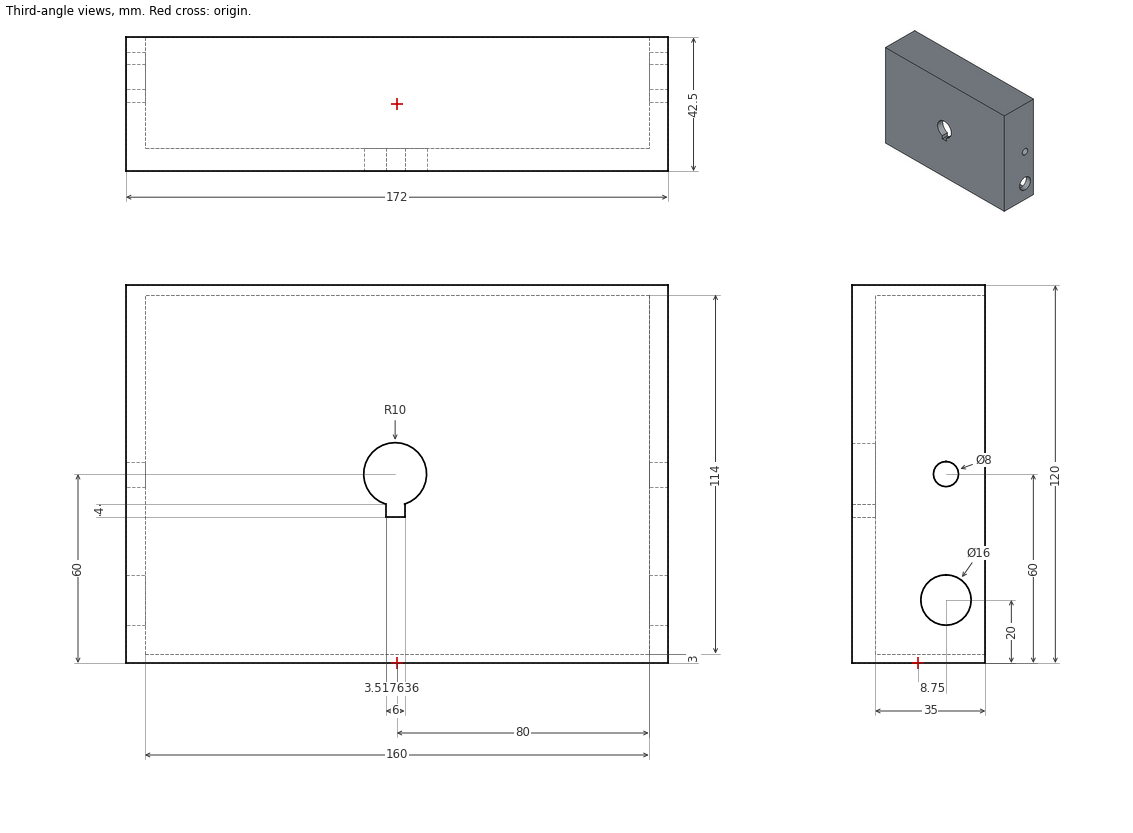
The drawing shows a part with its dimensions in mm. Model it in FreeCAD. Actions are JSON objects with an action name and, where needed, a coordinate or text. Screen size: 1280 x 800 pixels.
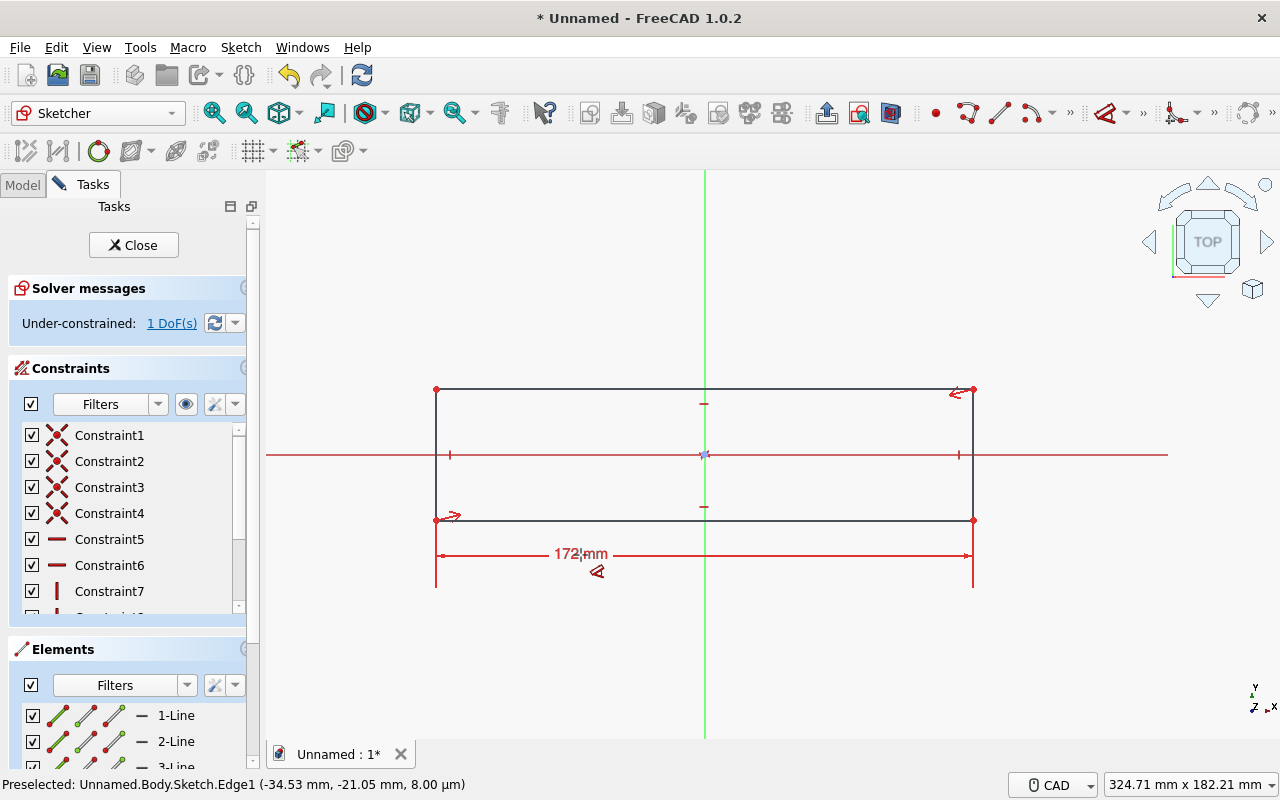
{"action": "left_click", "coordinate": [973, 481]}
{"action": "left_click", "coordinate": [1007, 425]}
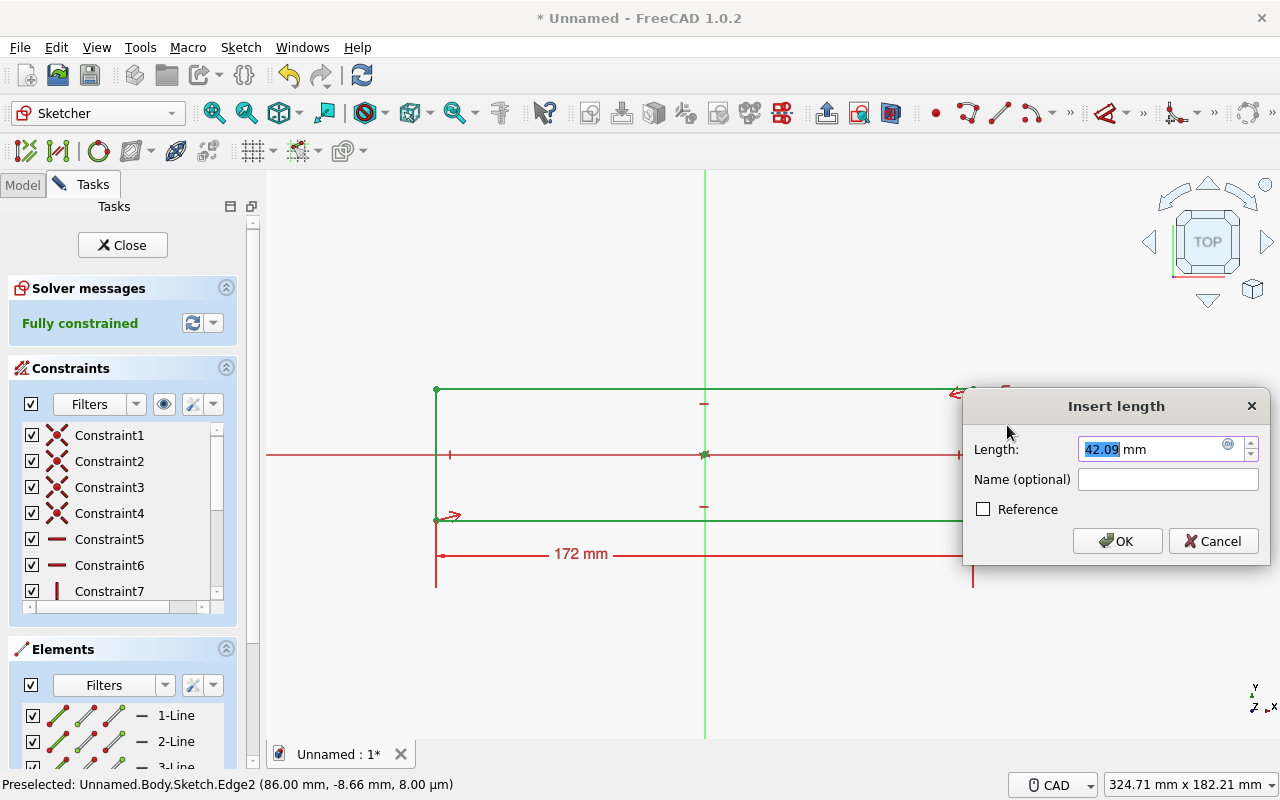
{"action": "type", "text": "42.5"}
{"action": "key", "text": "Return"}
{"action": "key", "text": "Escape"}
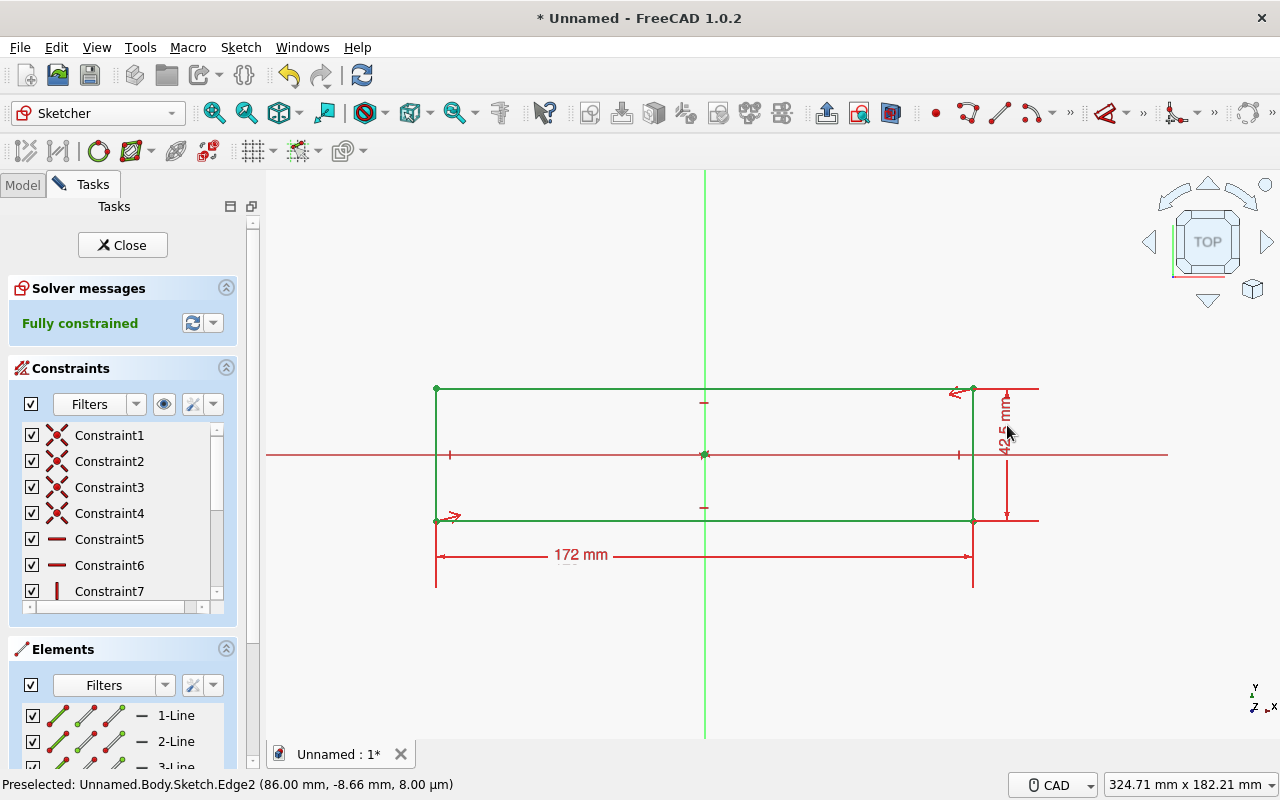
{"action": "left_click", "coordinate": [123, 245]}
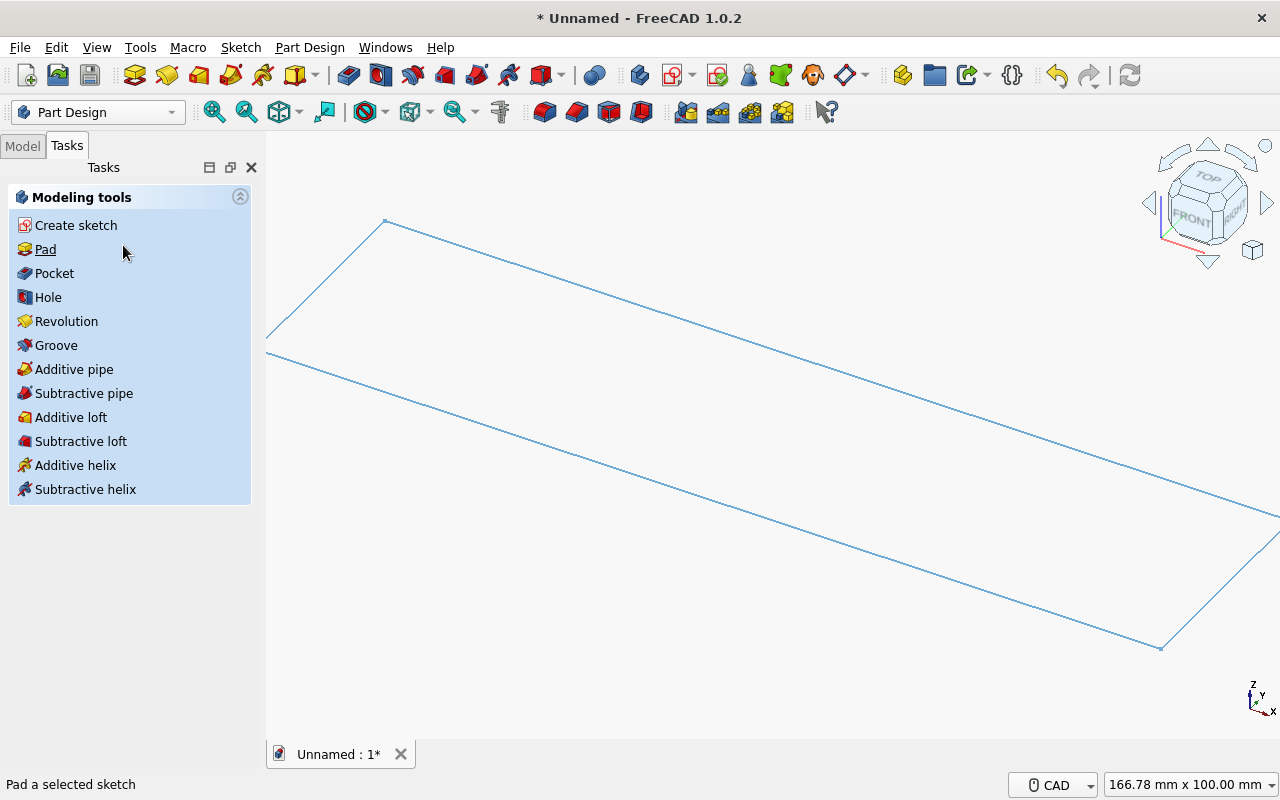
{"action": "left_click", "coordinate": [136, 76]}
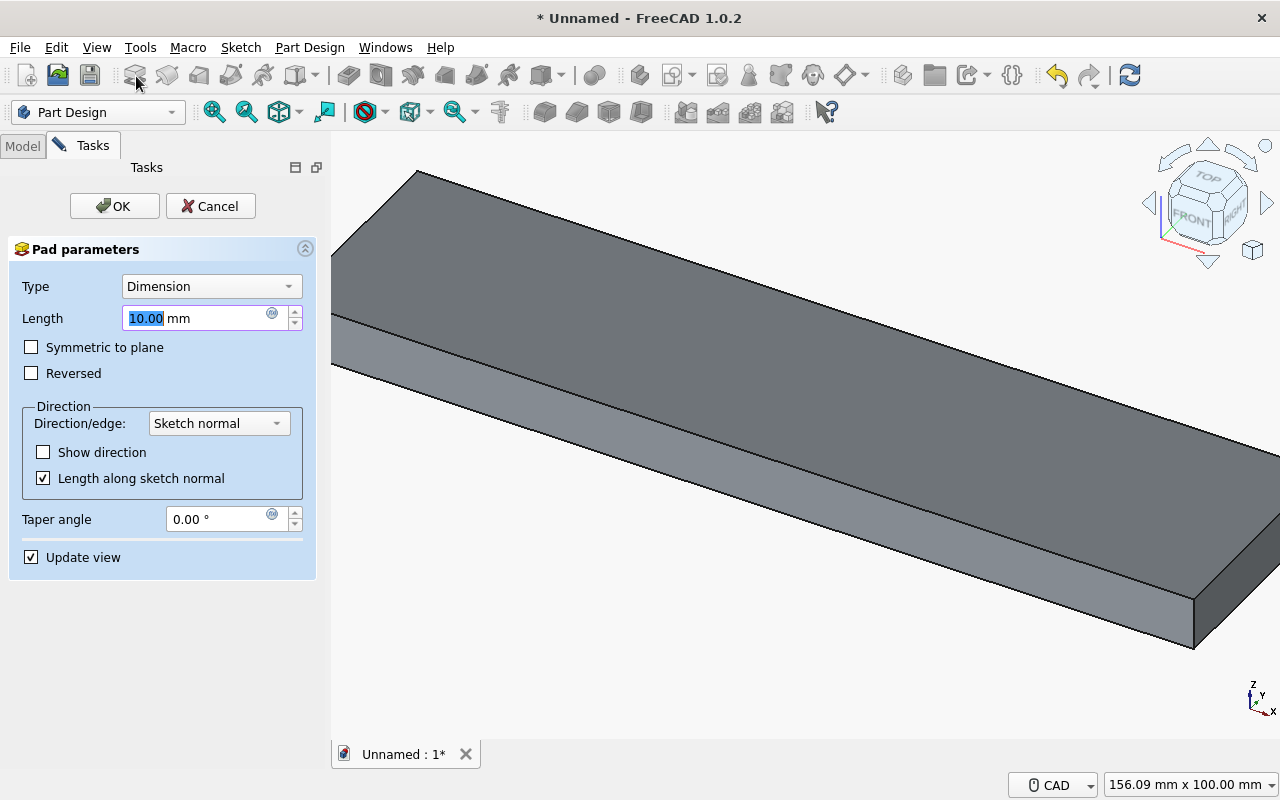
{"action": "type", "text": "120"}
{"action": "key", "text": "Tab"}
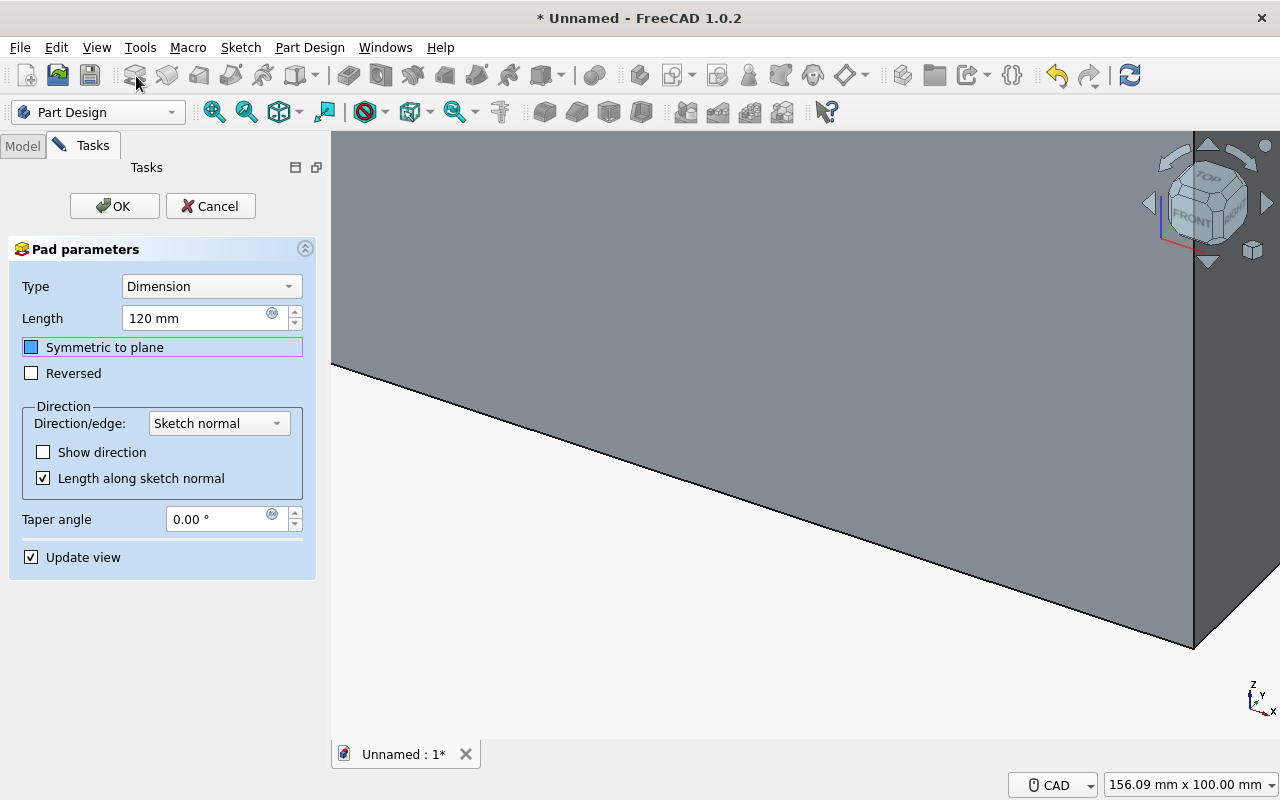
{"action": "left_click", "coordinate": [115, 206]}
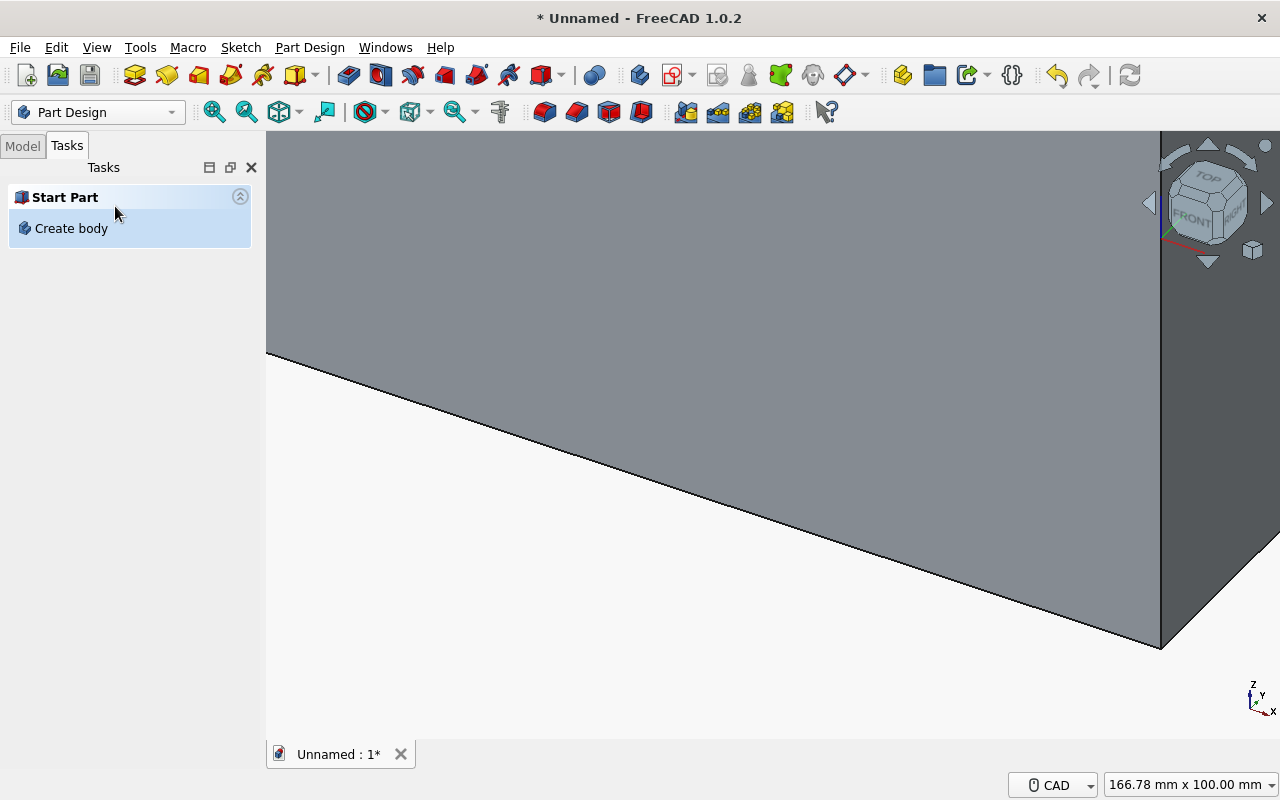
{"action": "left_click", "coordinate": [216, 112]}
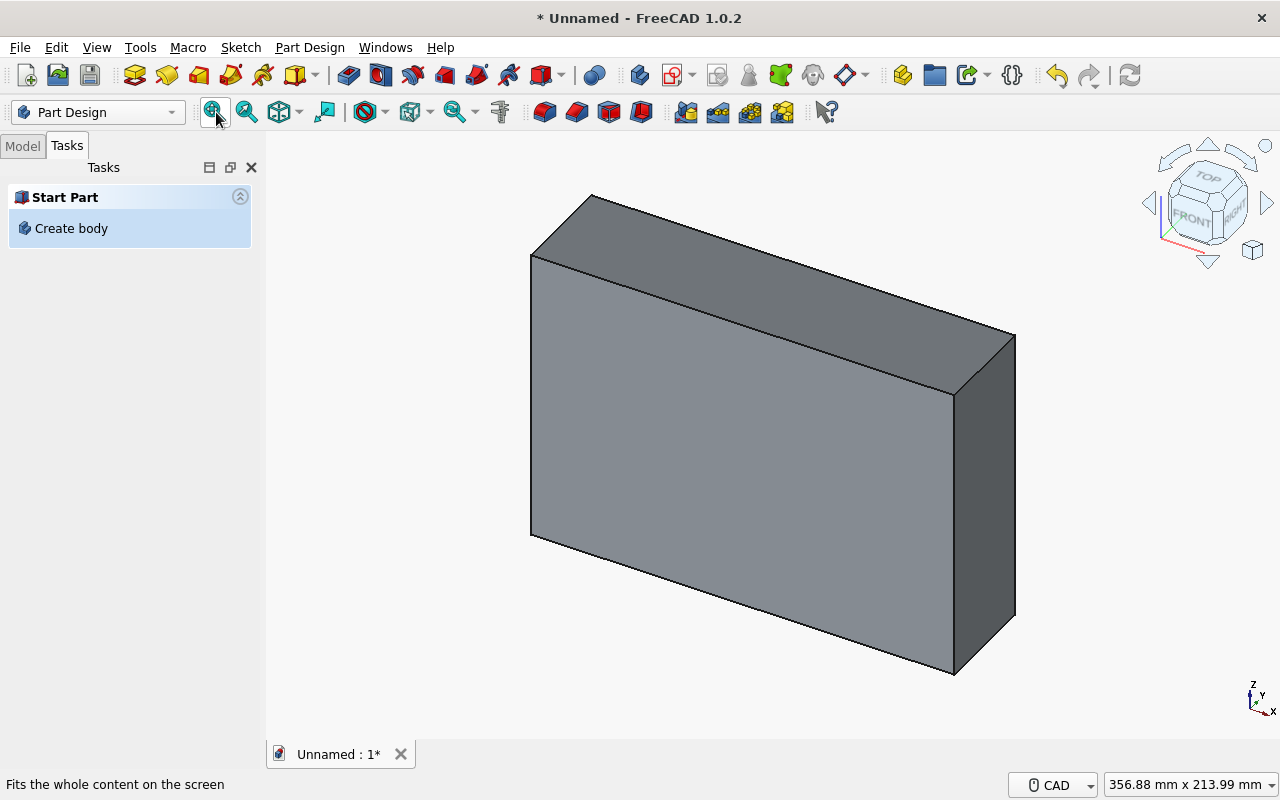
{"action": "key", "text": "4"}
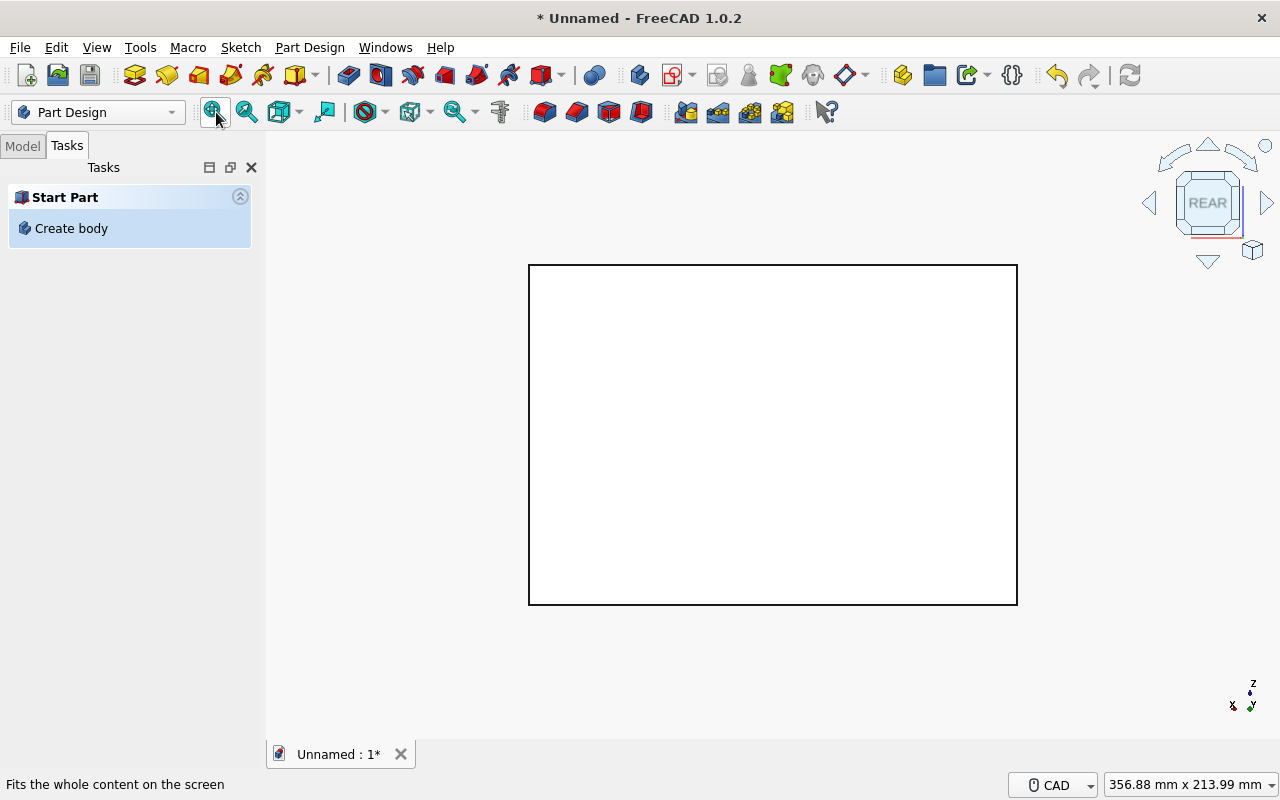
{"action": "left_click", "coordinate": [703, 434]}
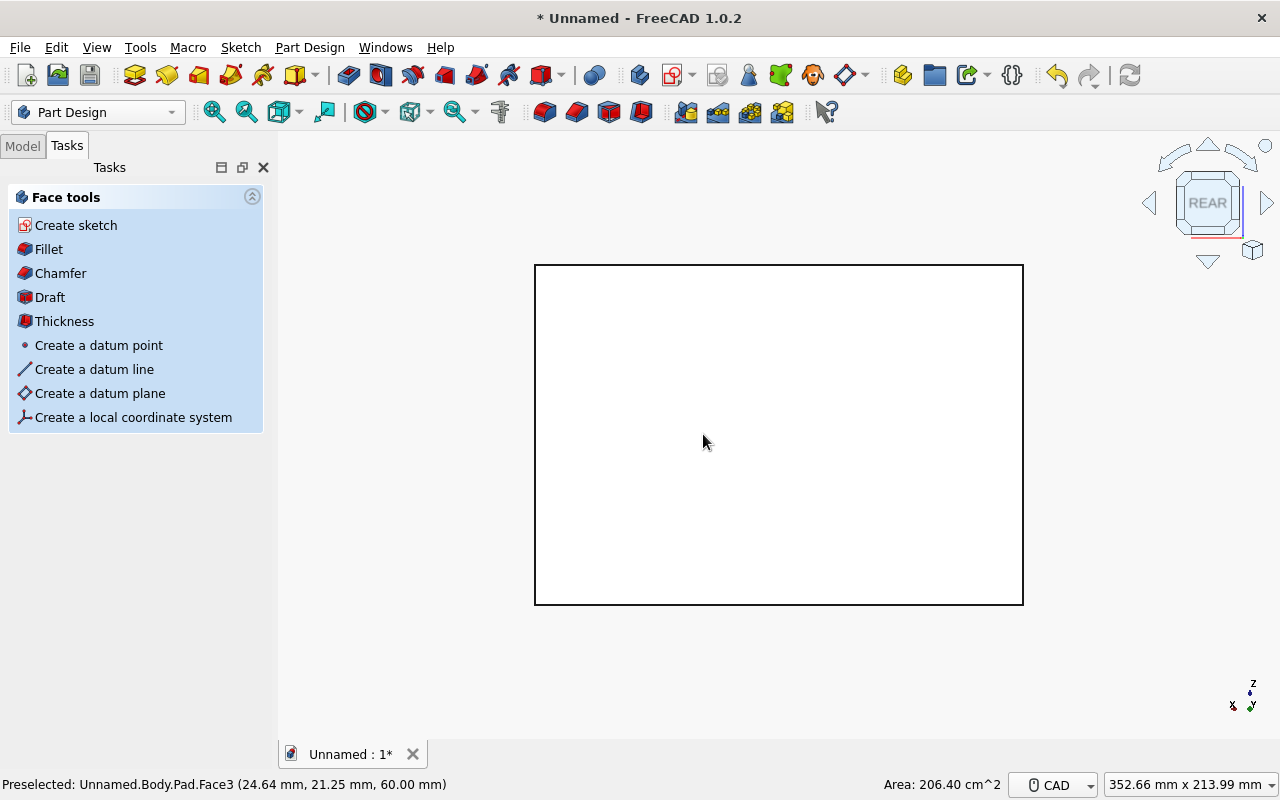
{"action": "left_click", "coordinate": [672, 76]}